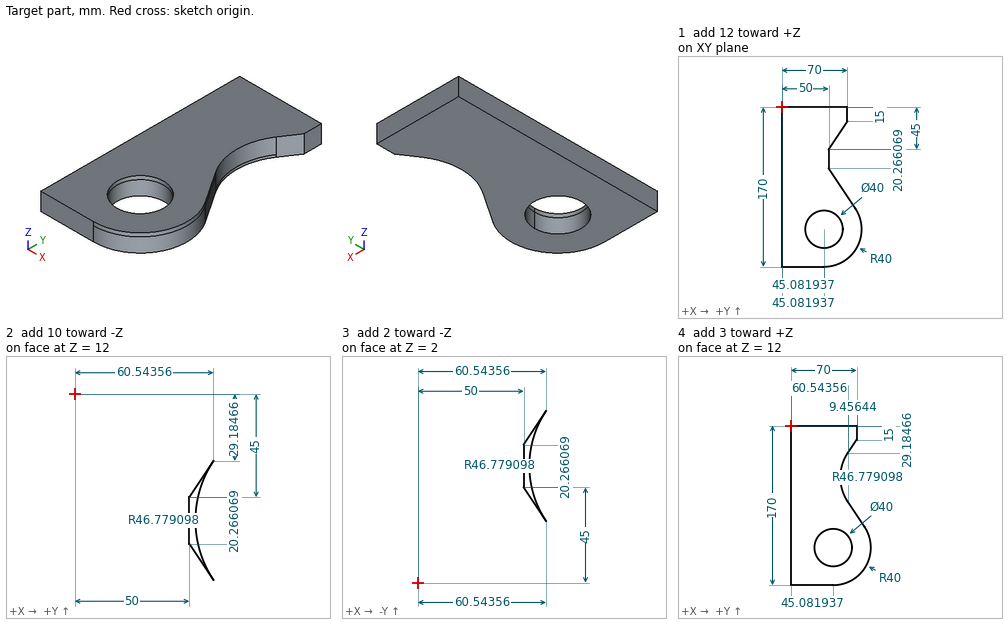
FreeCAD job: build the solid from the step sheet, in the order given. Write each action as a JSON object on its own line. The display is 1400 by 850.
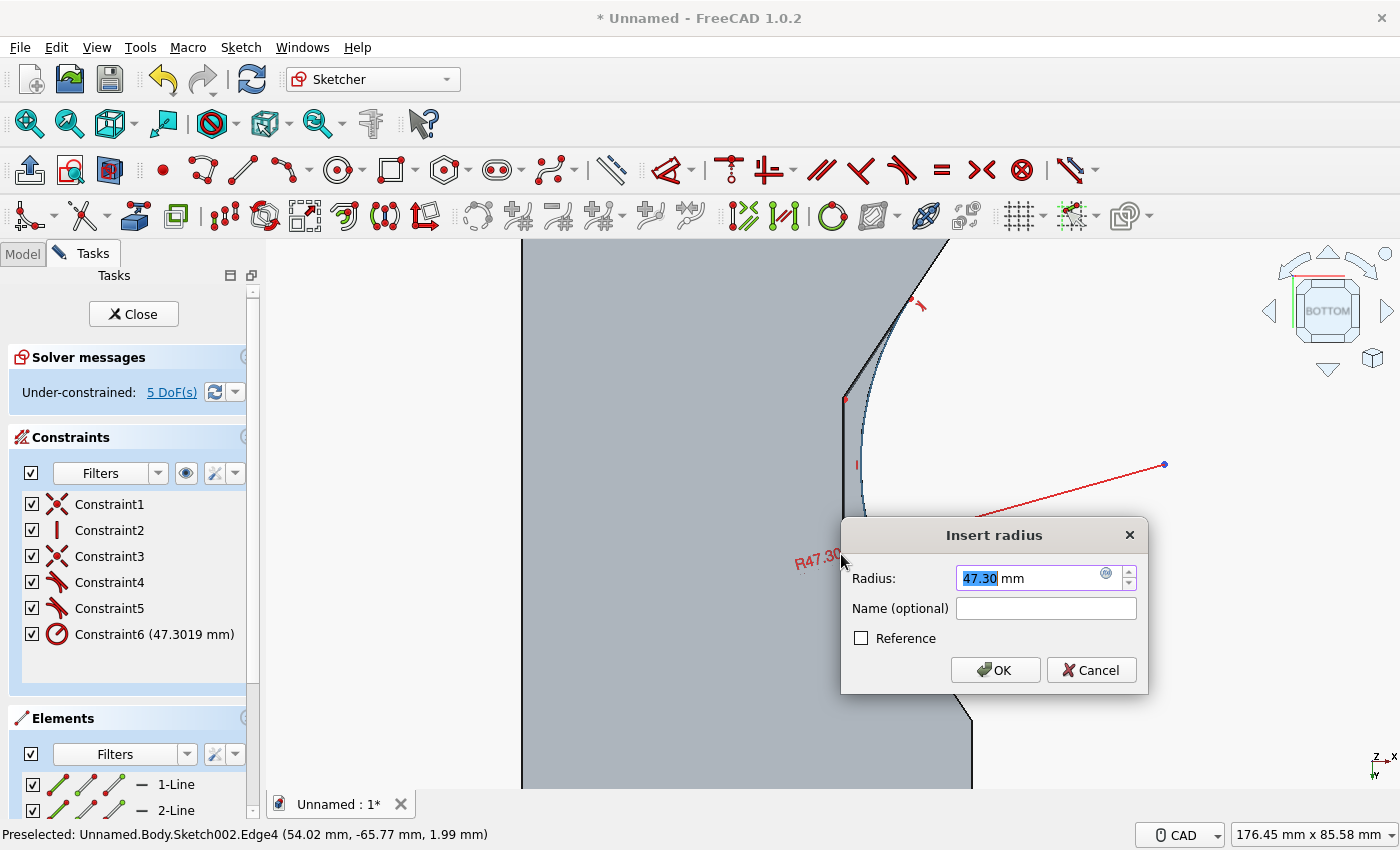
{"action": "type", "text": "46.779098"}
{"action": "key", "text": "Return"}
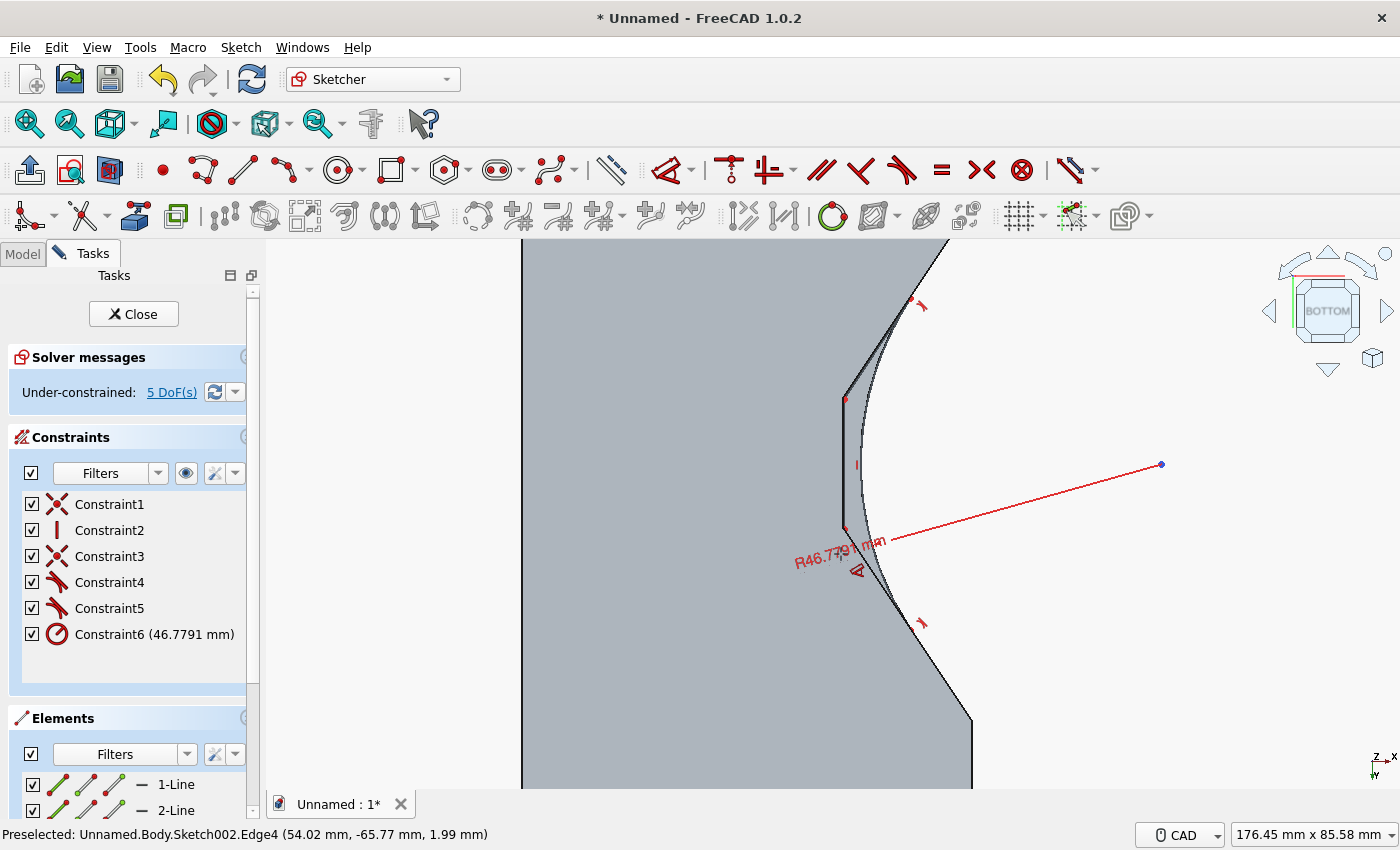
{"action": "left_click", "coordinate": [844, 399]}
{"action": "left_click", "coordinate": [683, 365]}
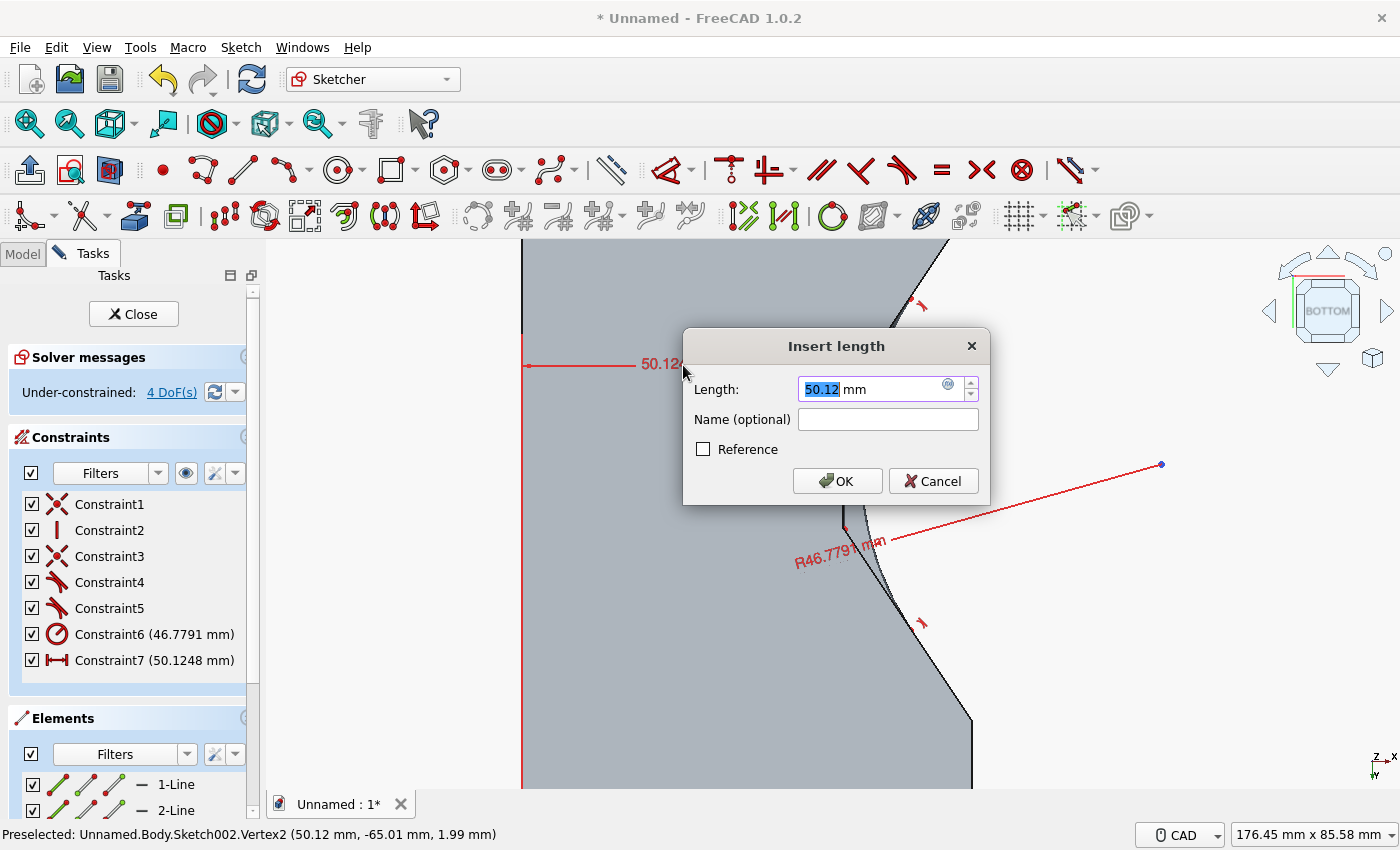
{"action": "type", "text": "50"}
{"action": "key", "text": "Return"}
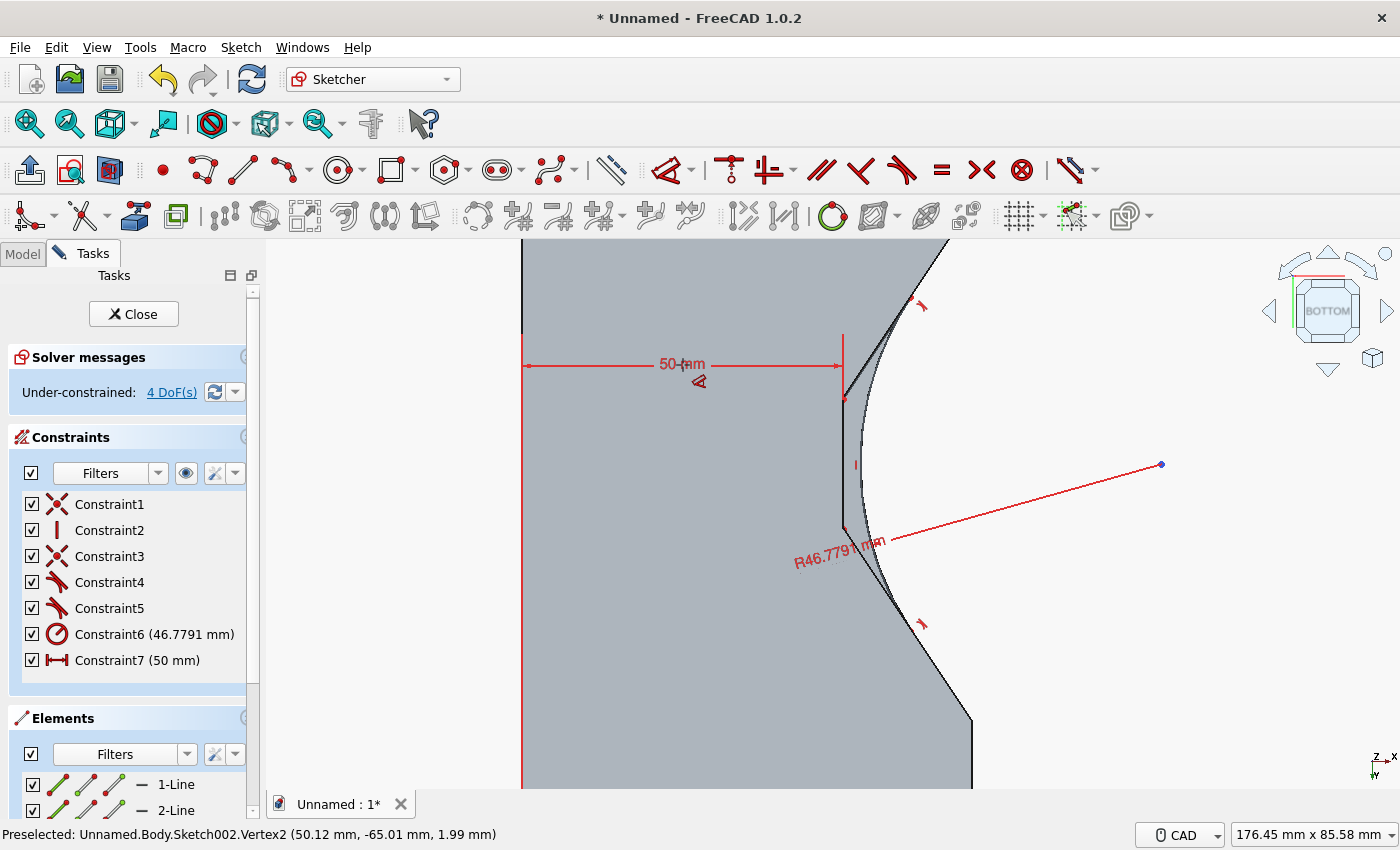
{"action": "left_click", "coordinate": [843, 529]}
{"action": "left_click", "coordinate": [488, 645]}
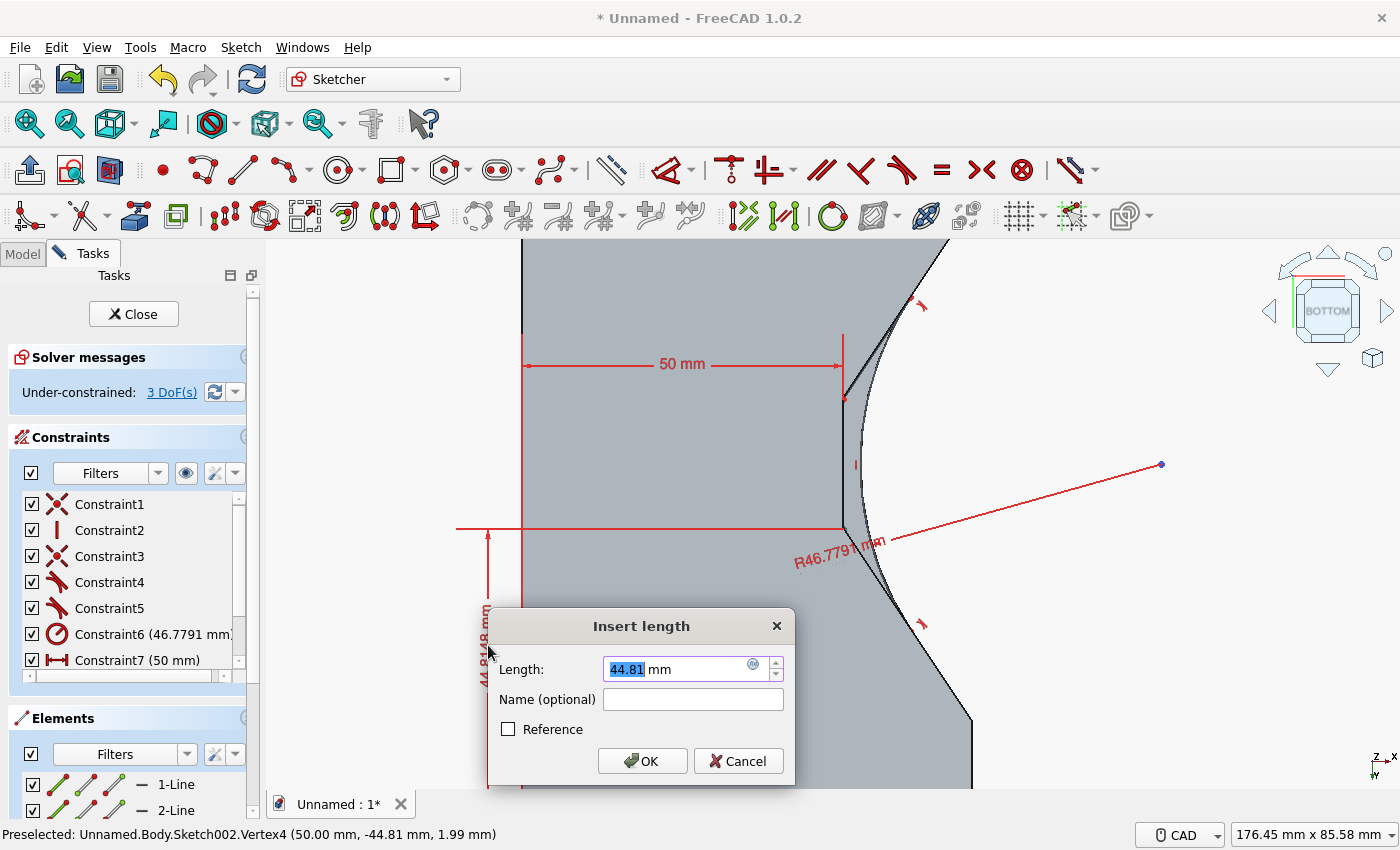
{"action": "type", "text": "45"}
{"action": "key", "text": "Return"}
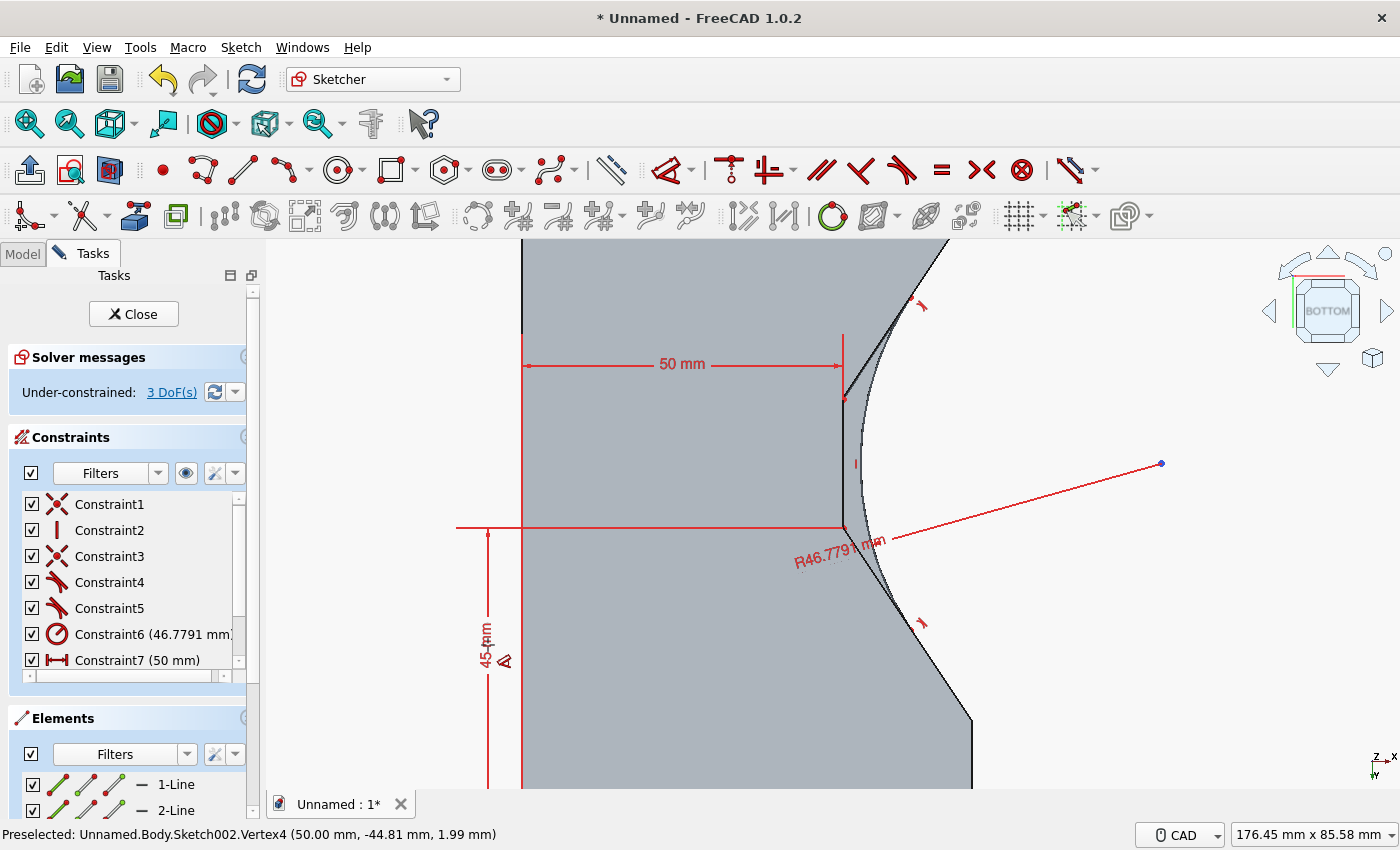
{"action": "left_click", "coordinate": [843, 438]}
{"action": "left_click", "coordinate": [877, 464]}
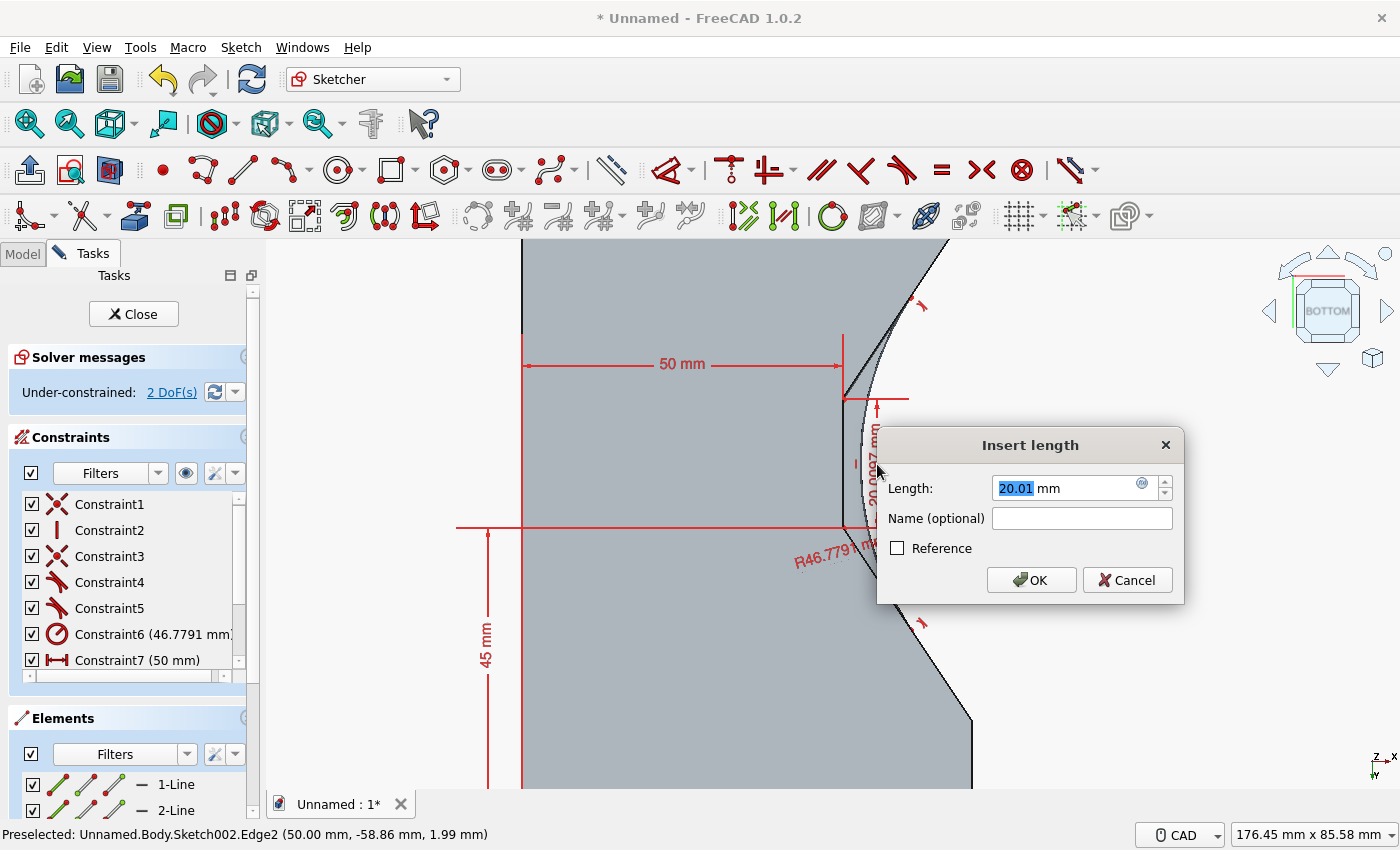
{"action": "type", "text": "20.266069"}
{"action": "key", "text": "Return"}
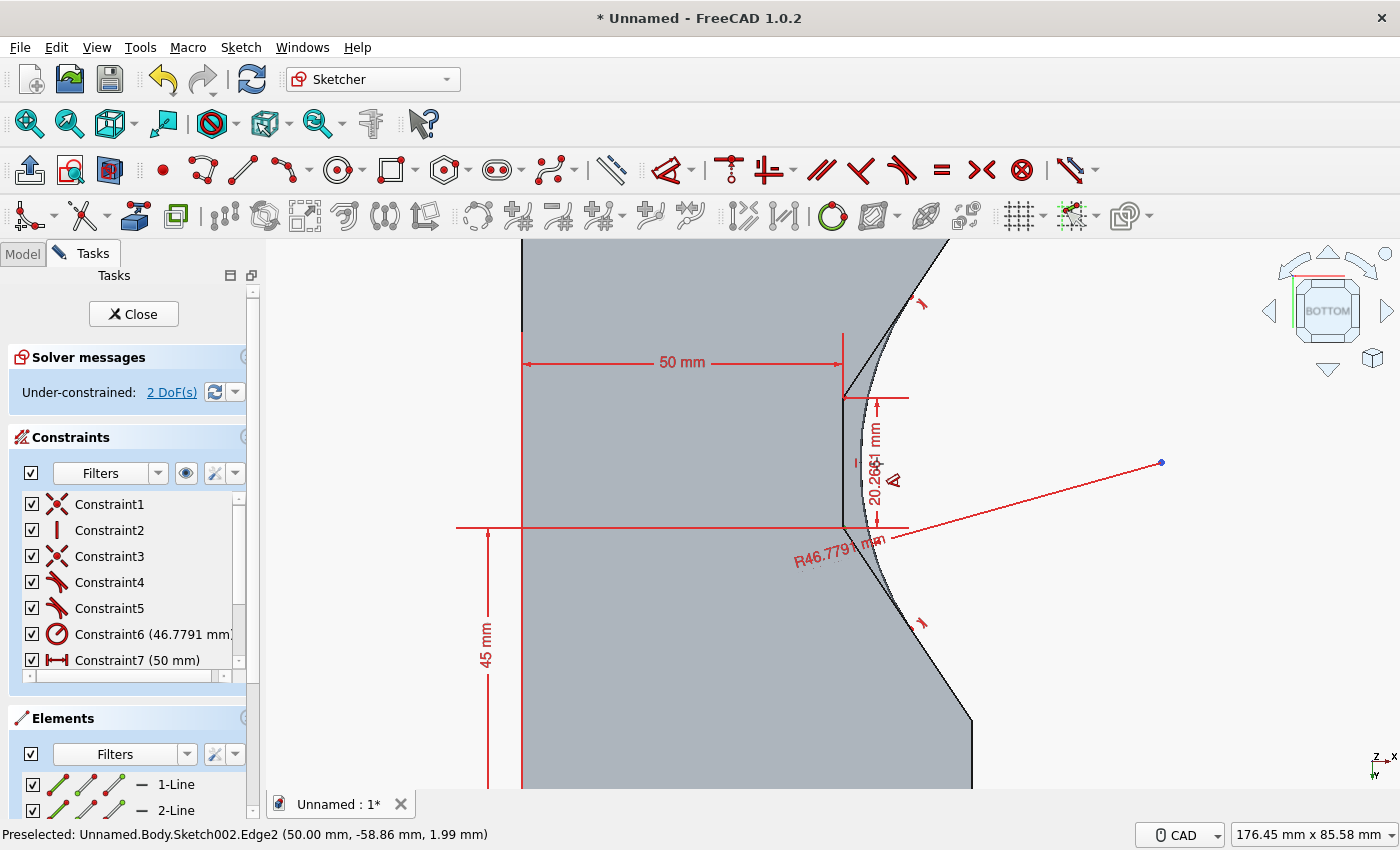
{"action": "left_click", "coordinate": [911, 296]}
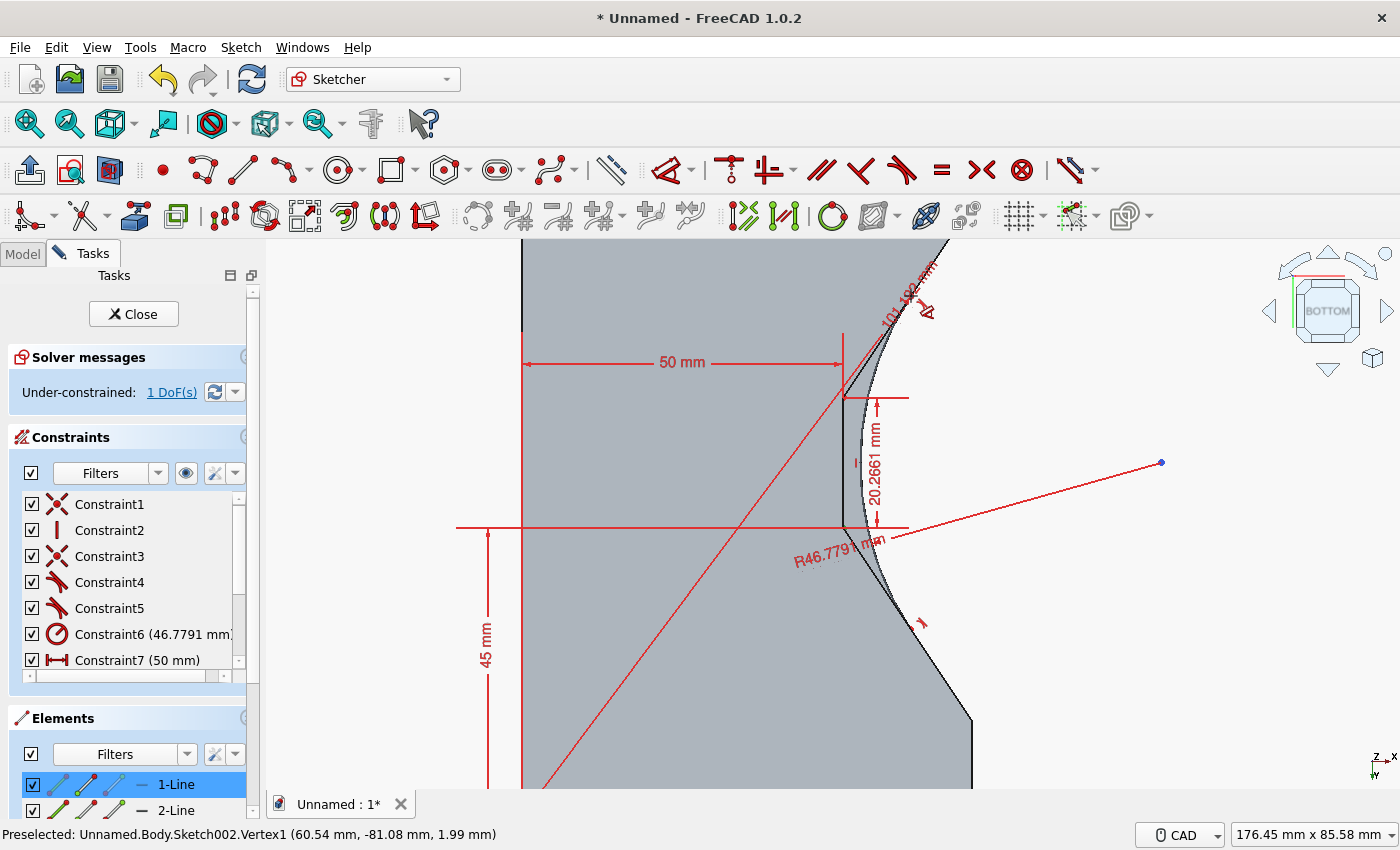
{"action": "key", "text": "Escape"}
{"action": "key", "text": "Escape"}